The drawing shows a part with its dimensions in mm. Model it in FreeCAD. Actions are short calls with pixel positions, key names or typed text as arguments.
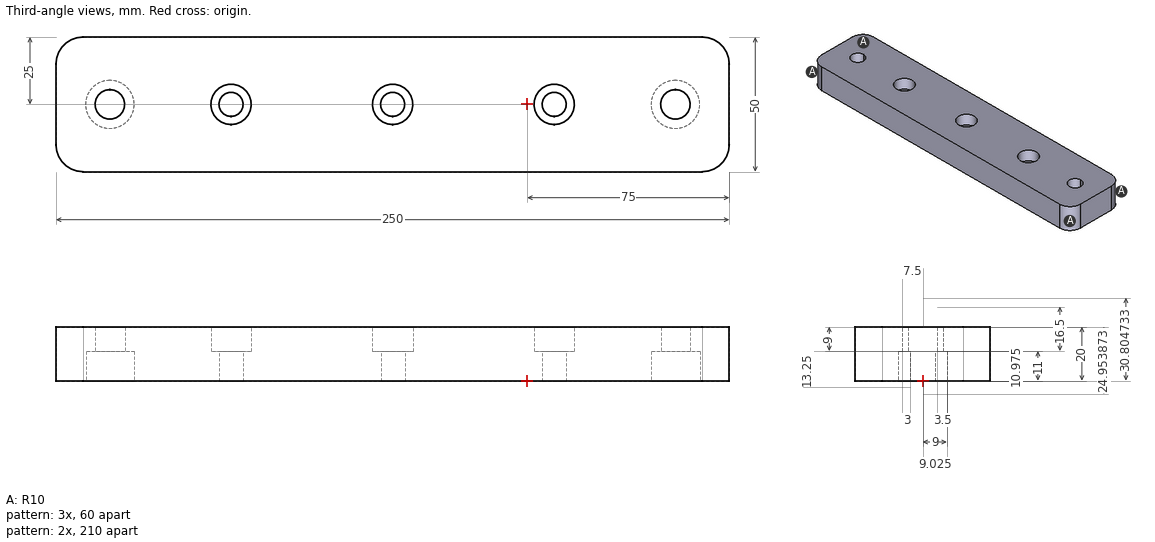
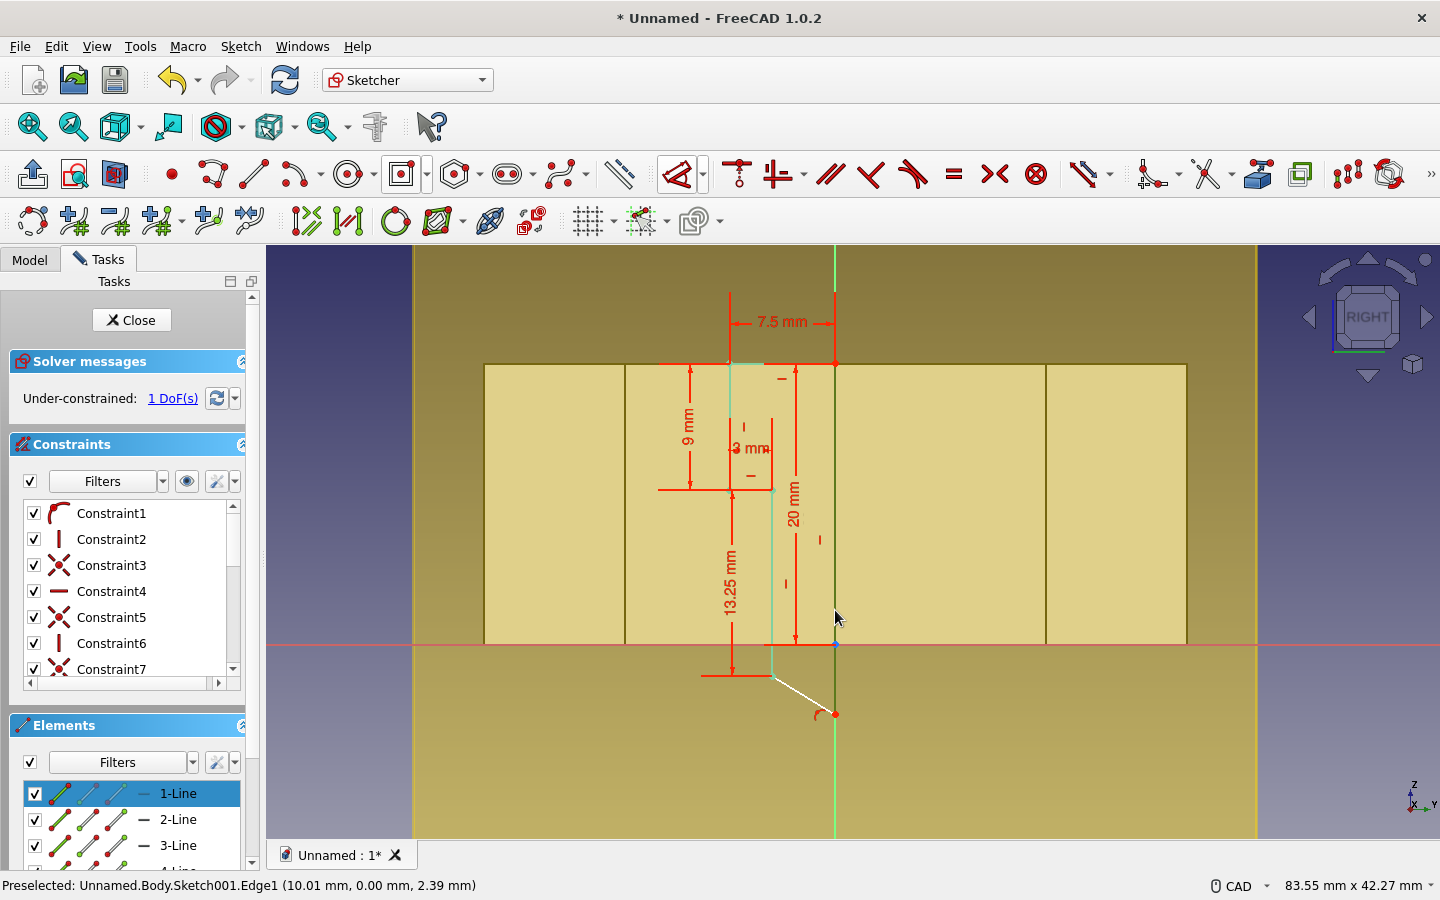
key(i)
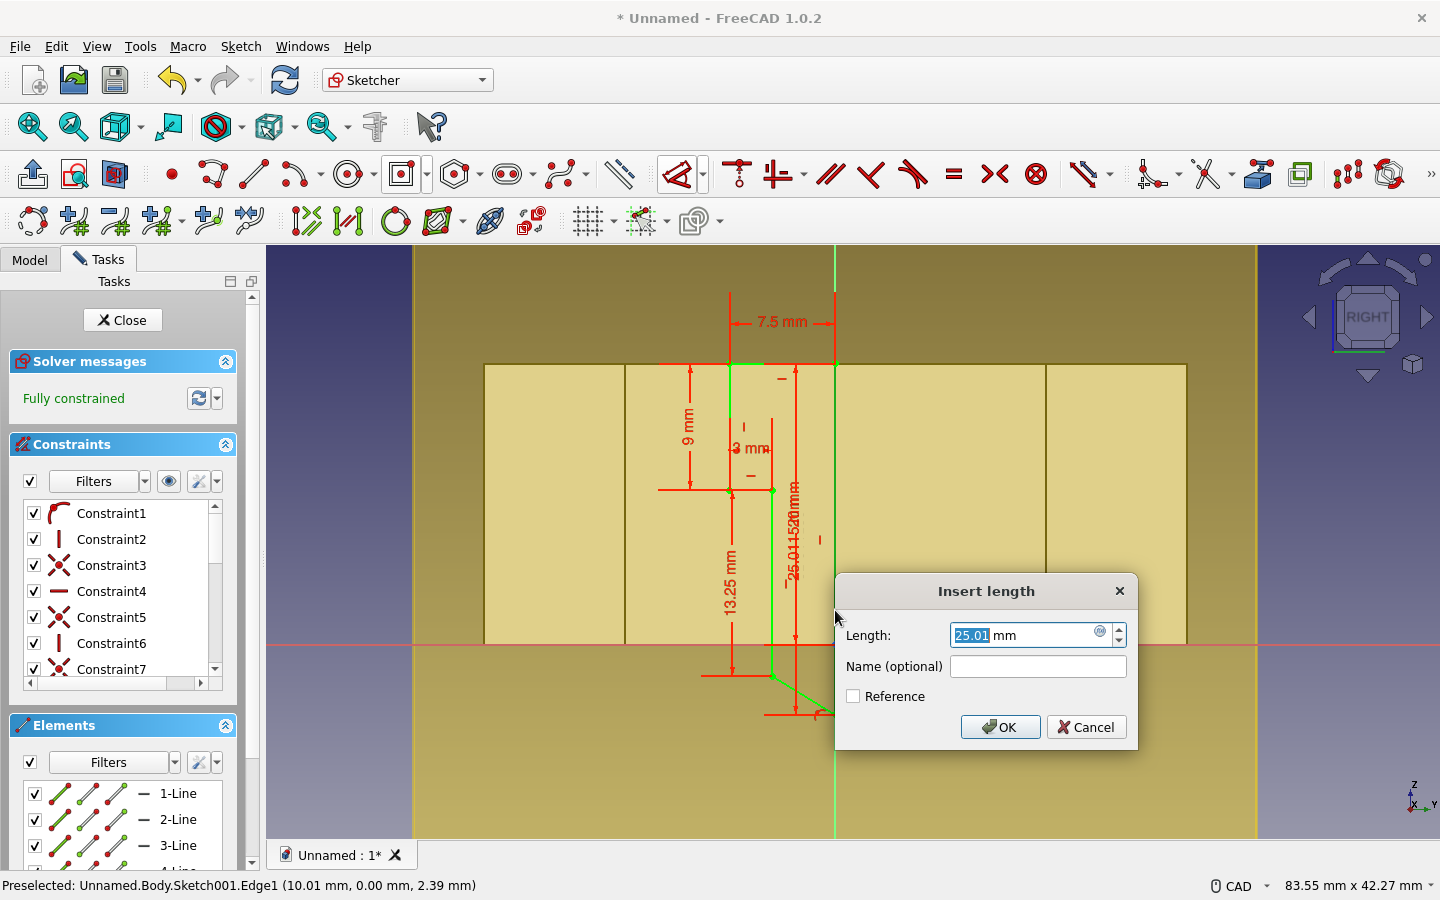
text(24.953873)
key(Return)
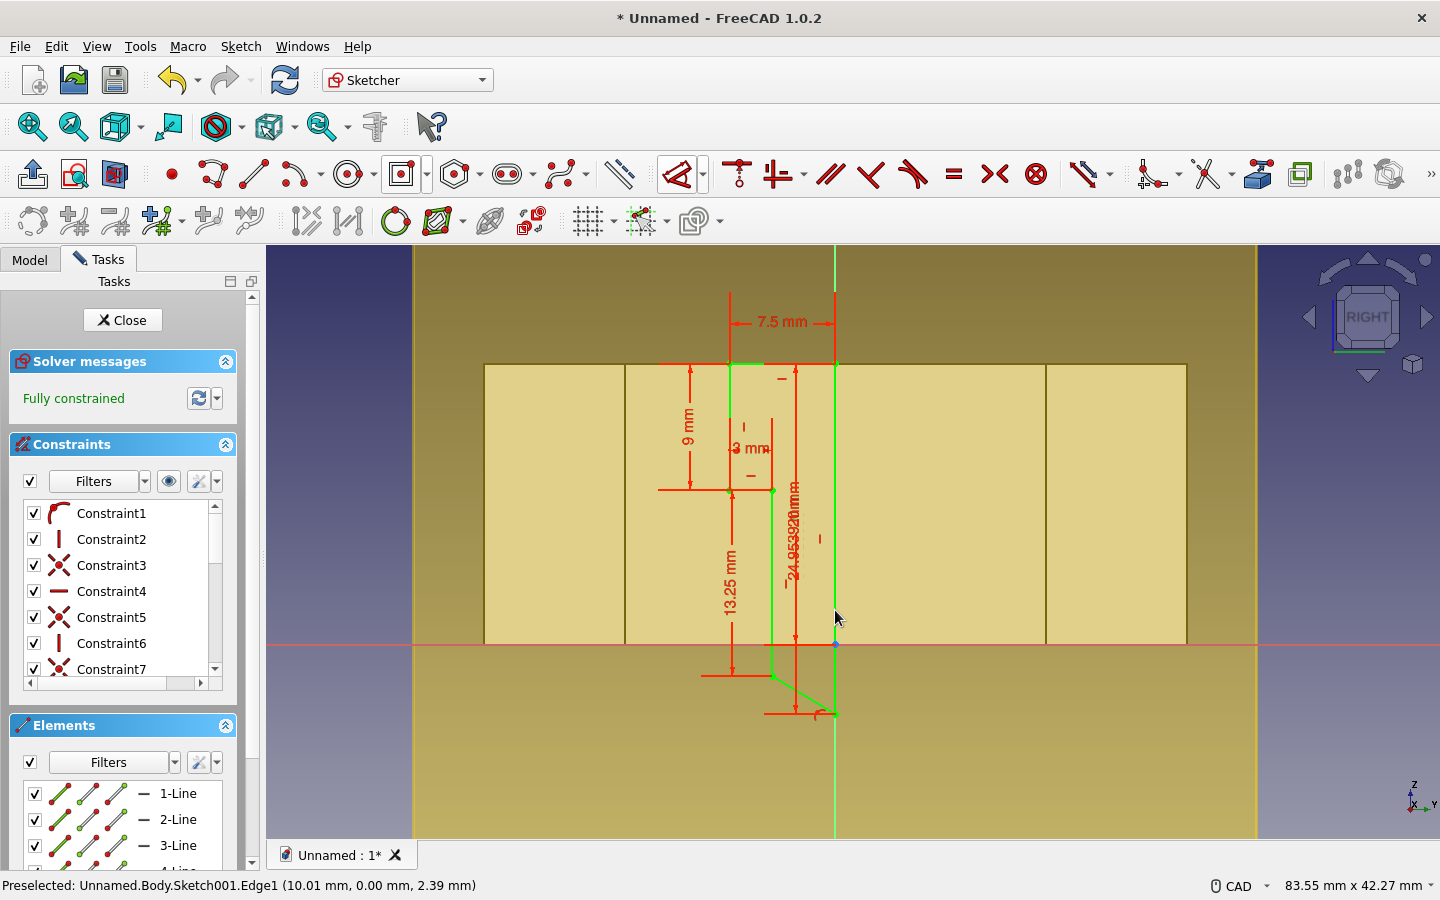
click(123, 320)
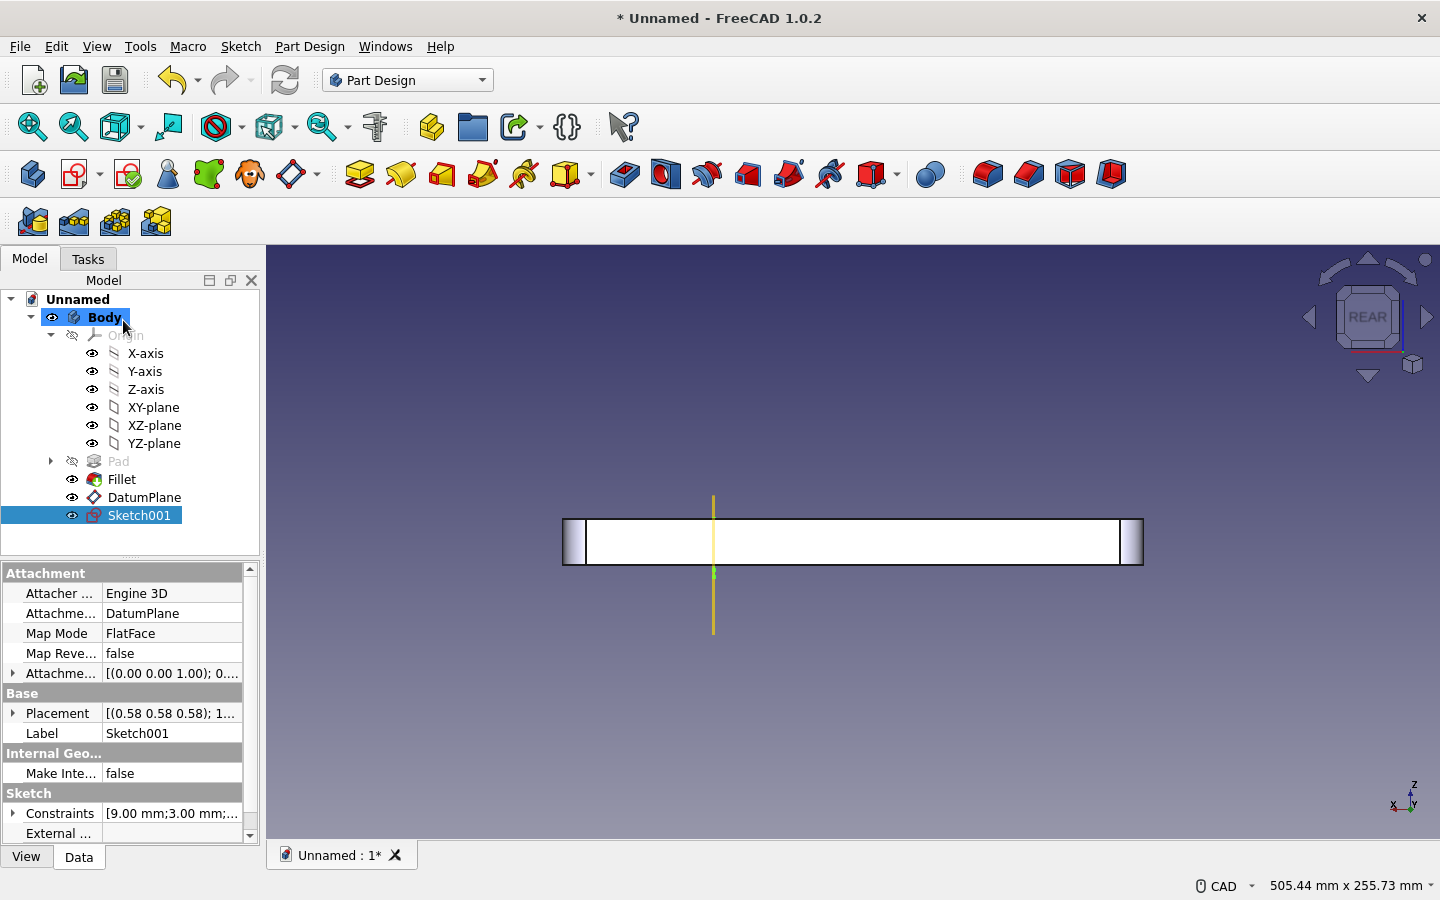
click(707, 174)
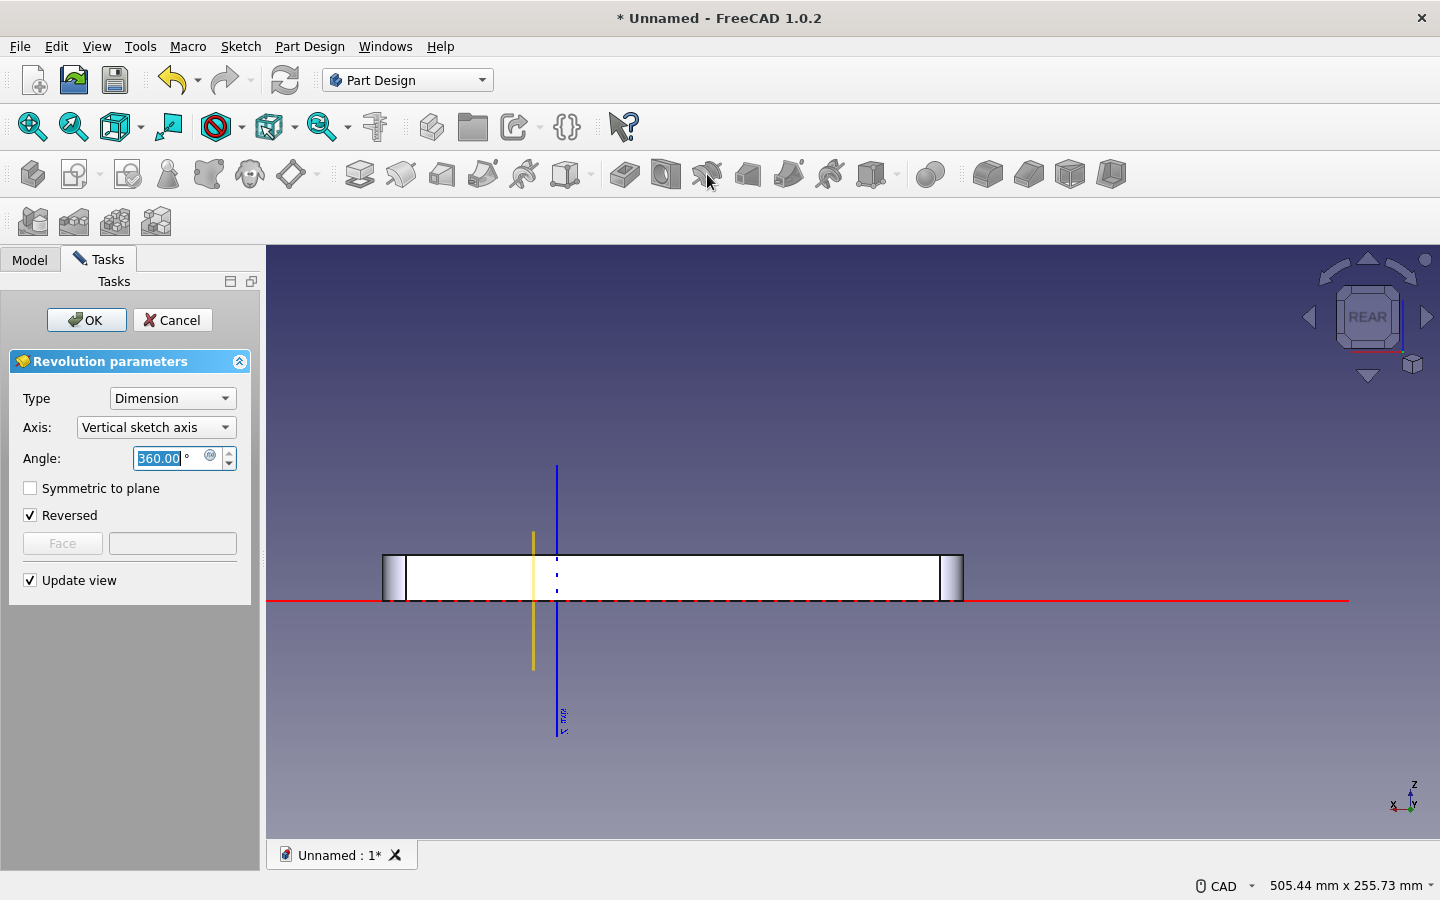
click(87, 320)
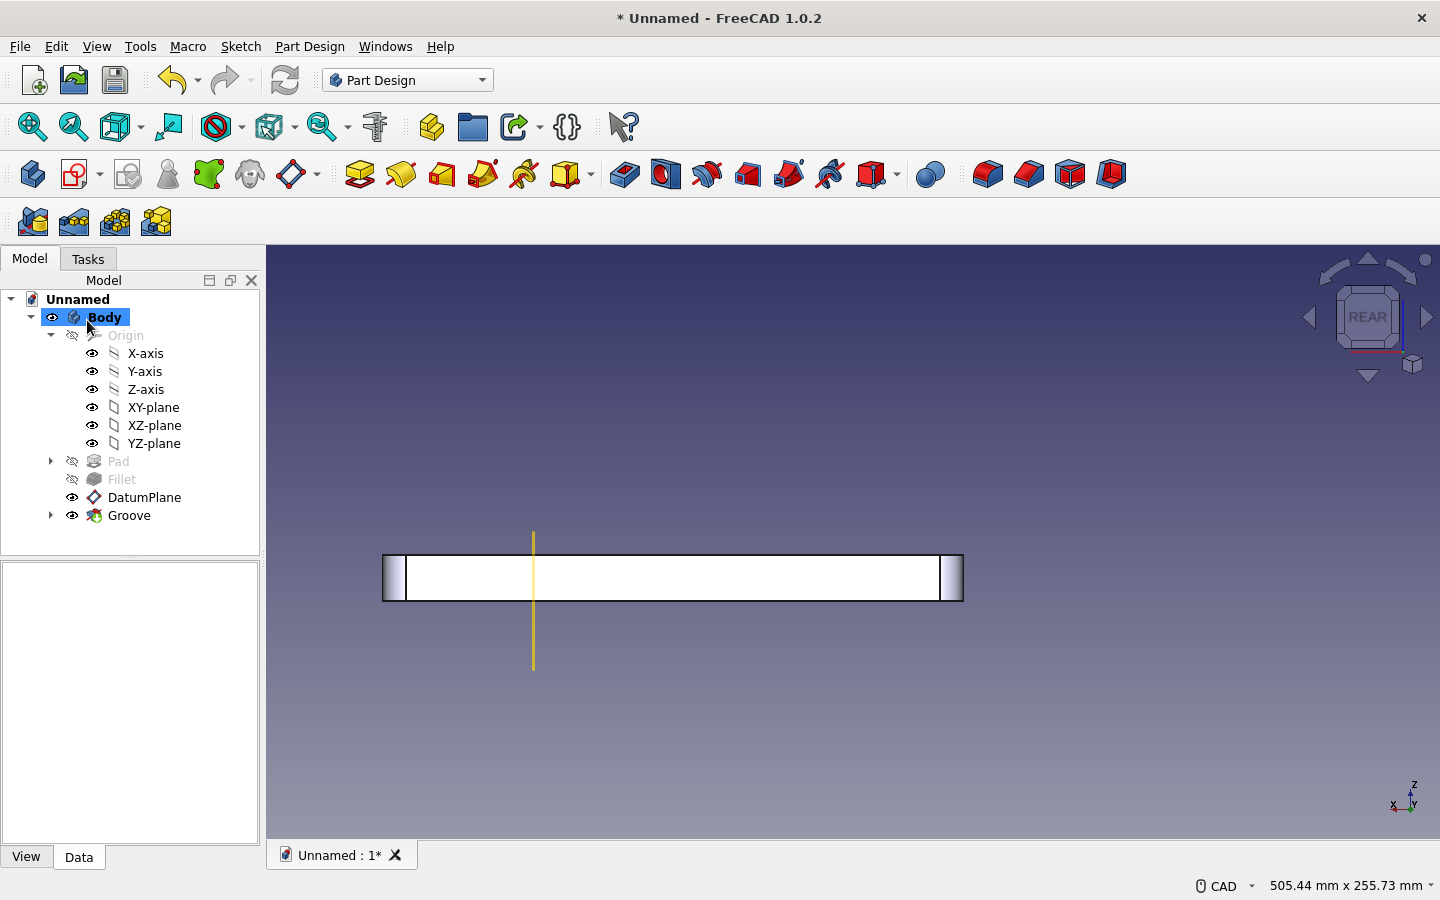
click(117, 497)
key(space)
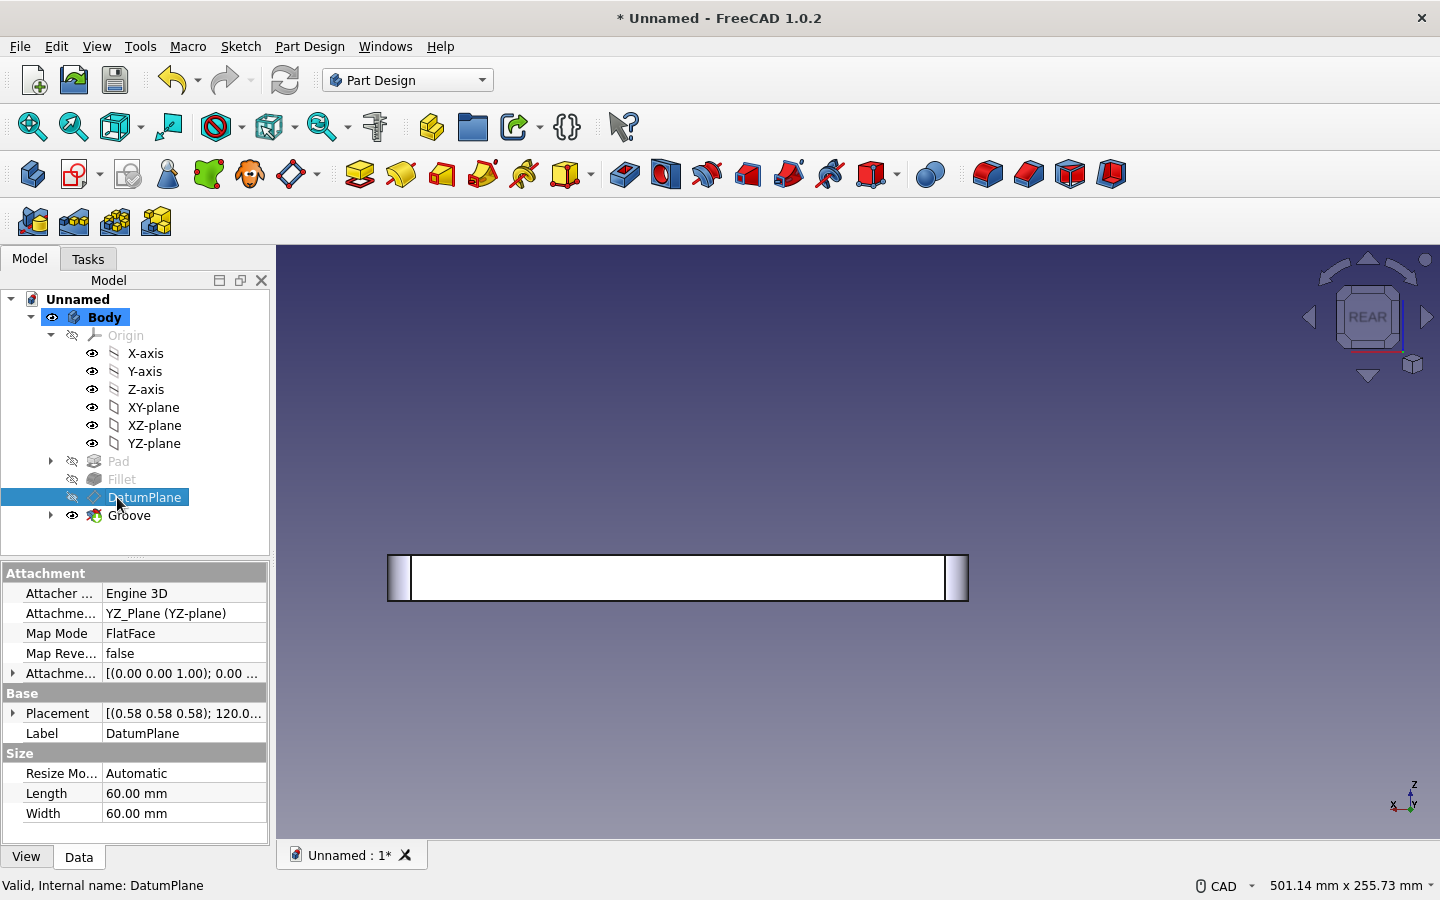
click(117, 515)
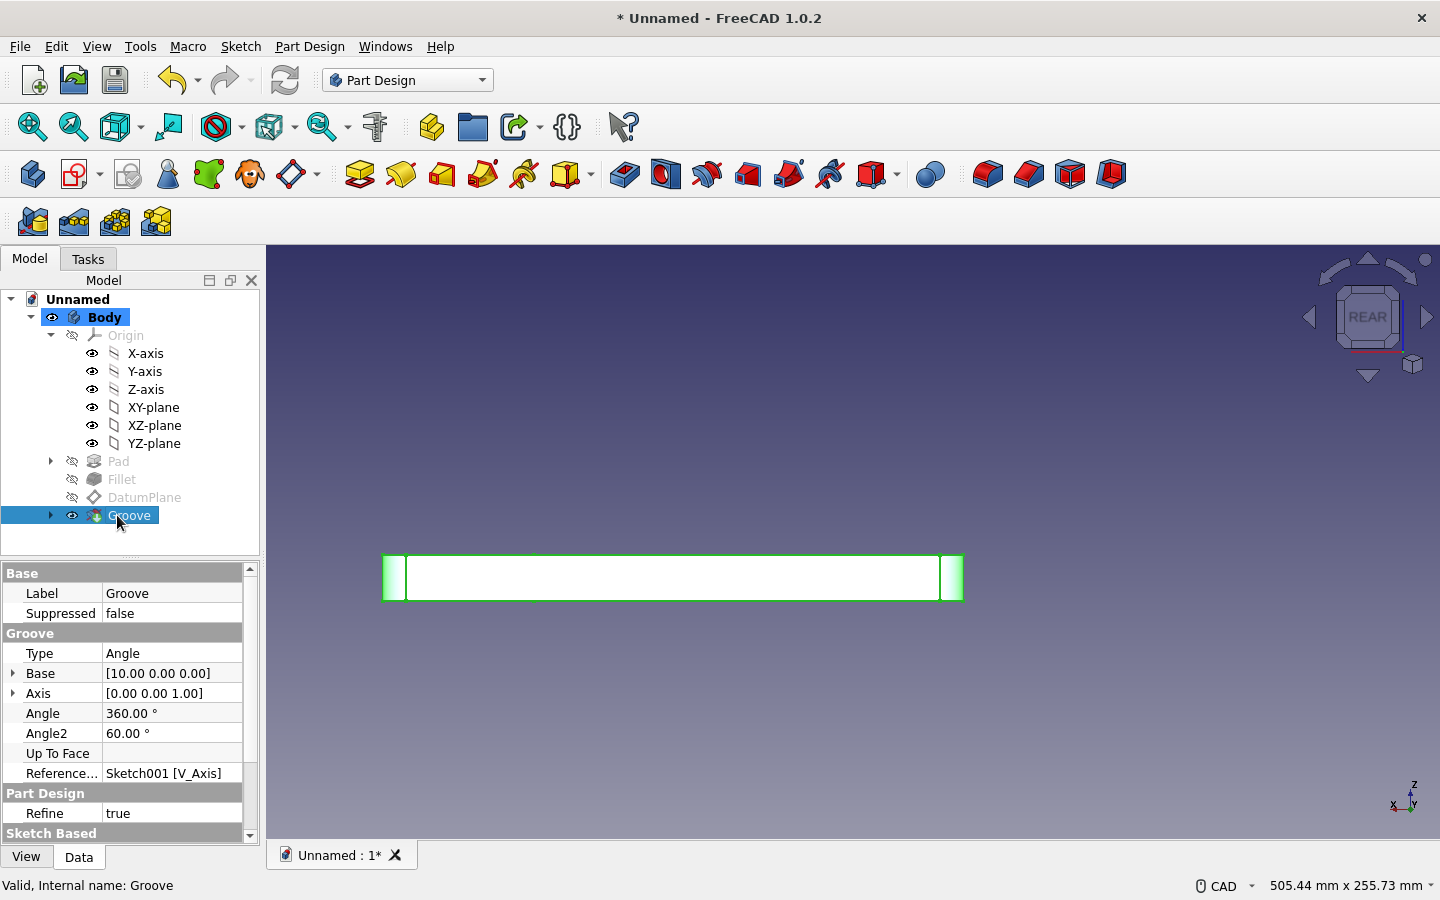
click(74, 222)